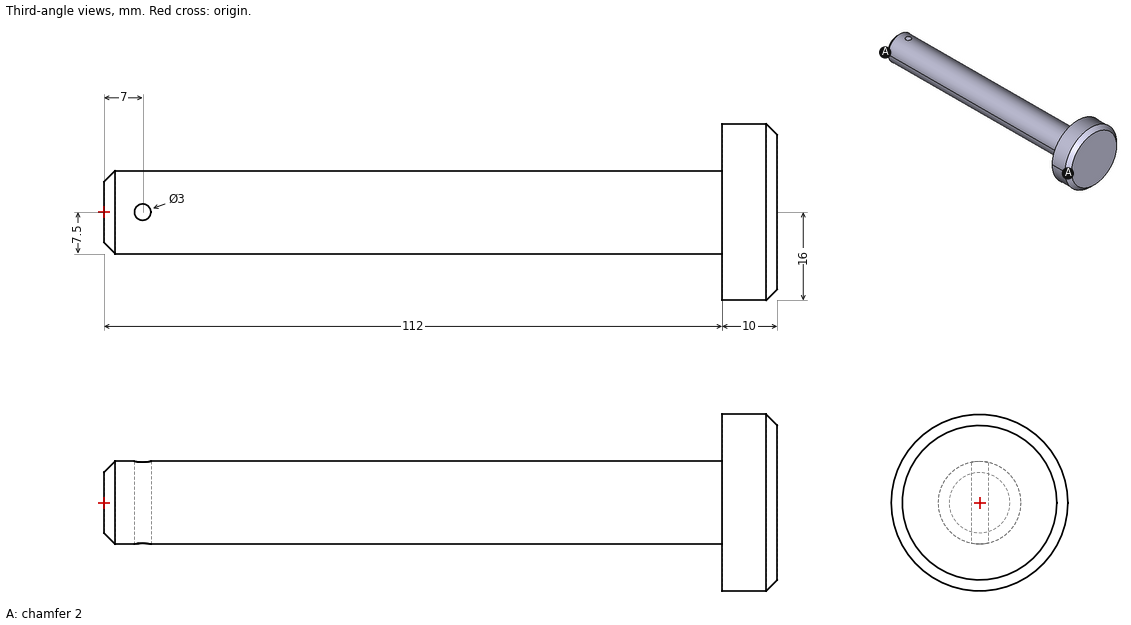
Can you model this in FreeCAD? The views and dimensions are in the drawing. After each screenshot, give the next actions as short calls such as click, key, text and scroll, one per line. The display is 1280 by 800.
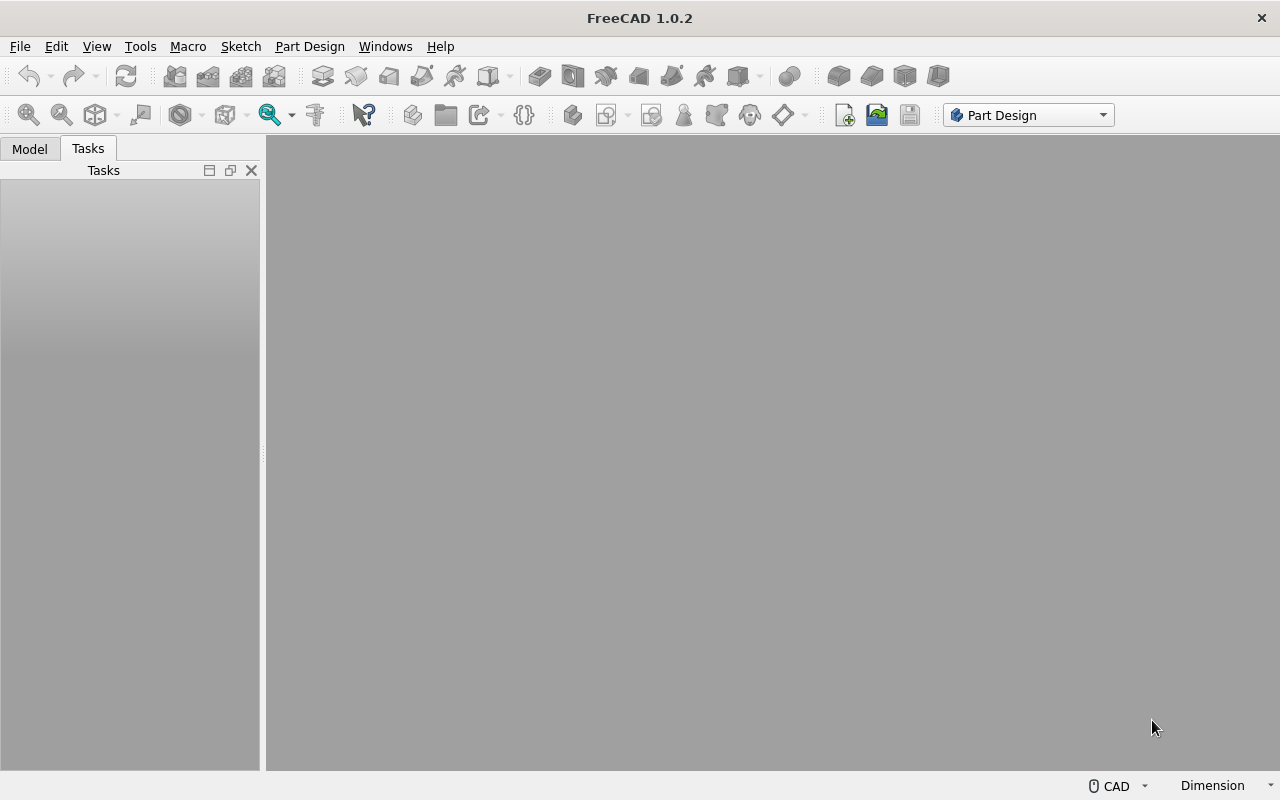
click(844, 116)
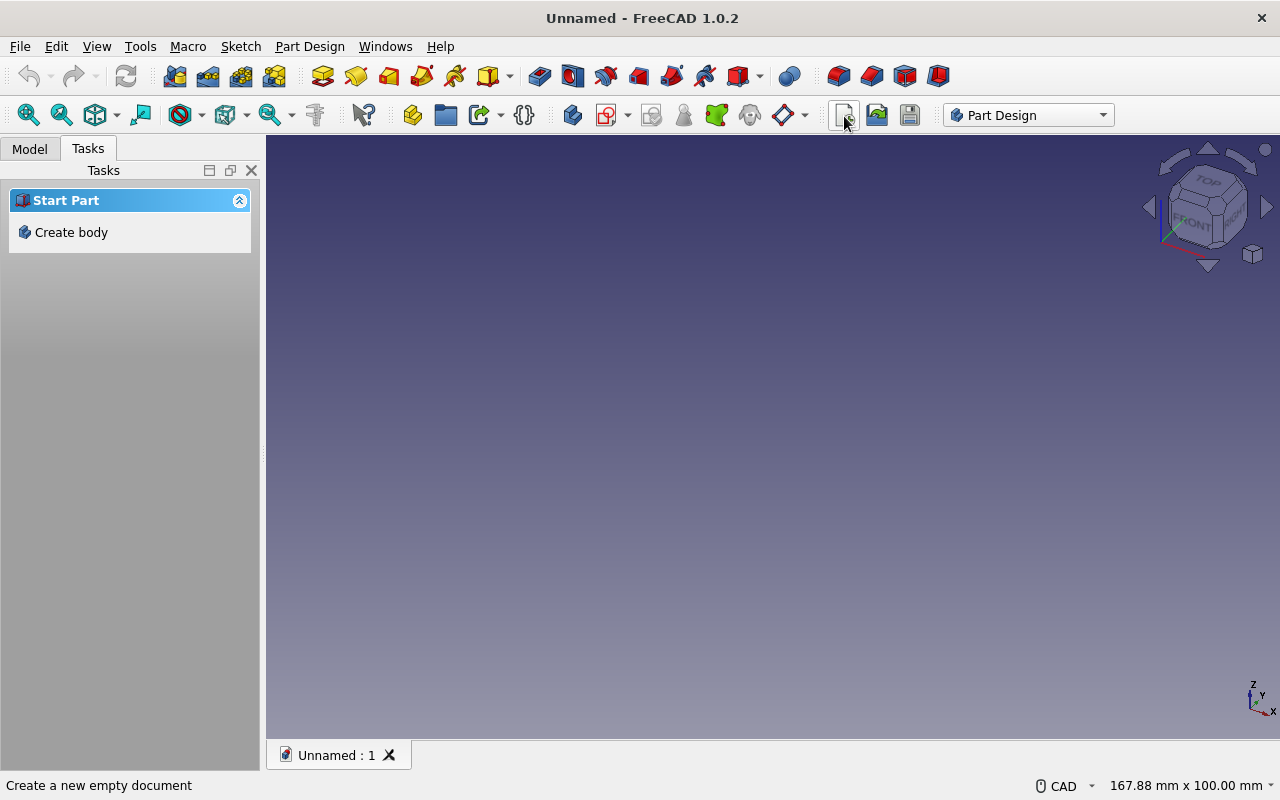
click(606, 116)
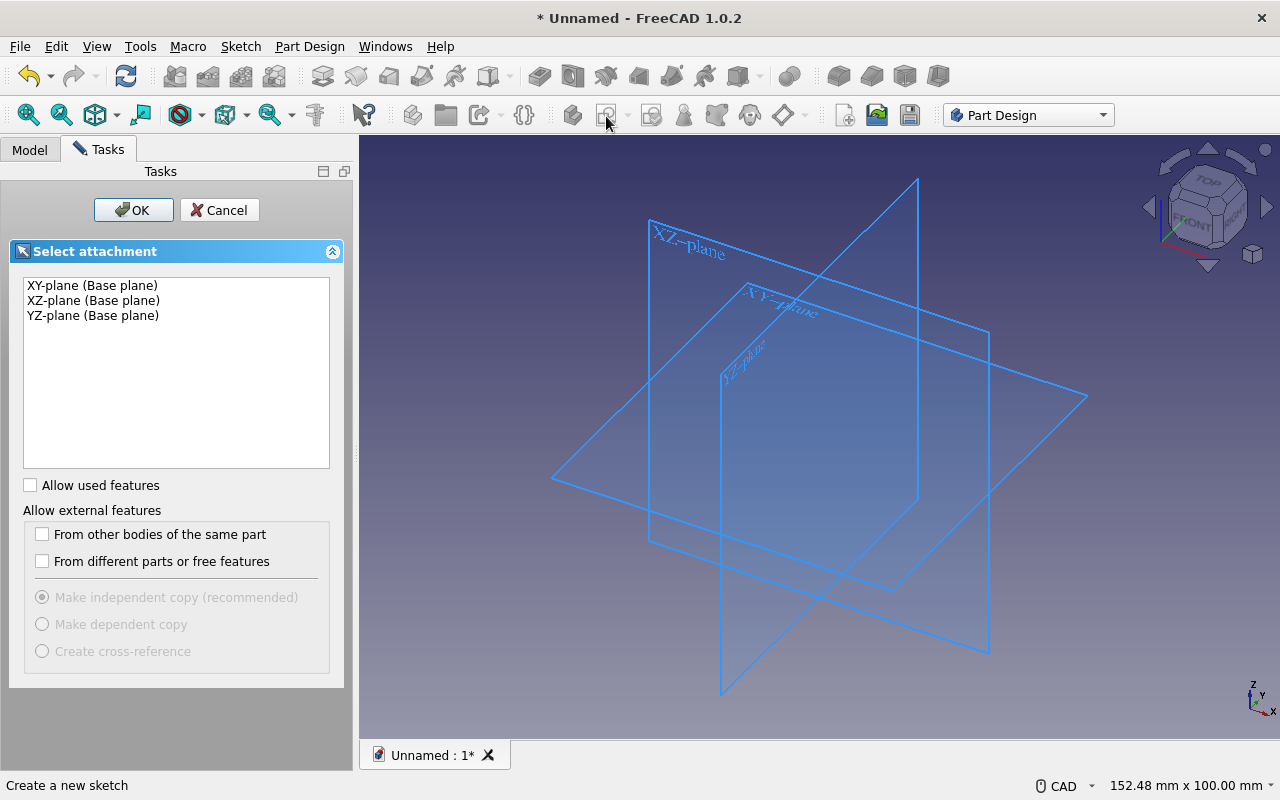
click(84, 286)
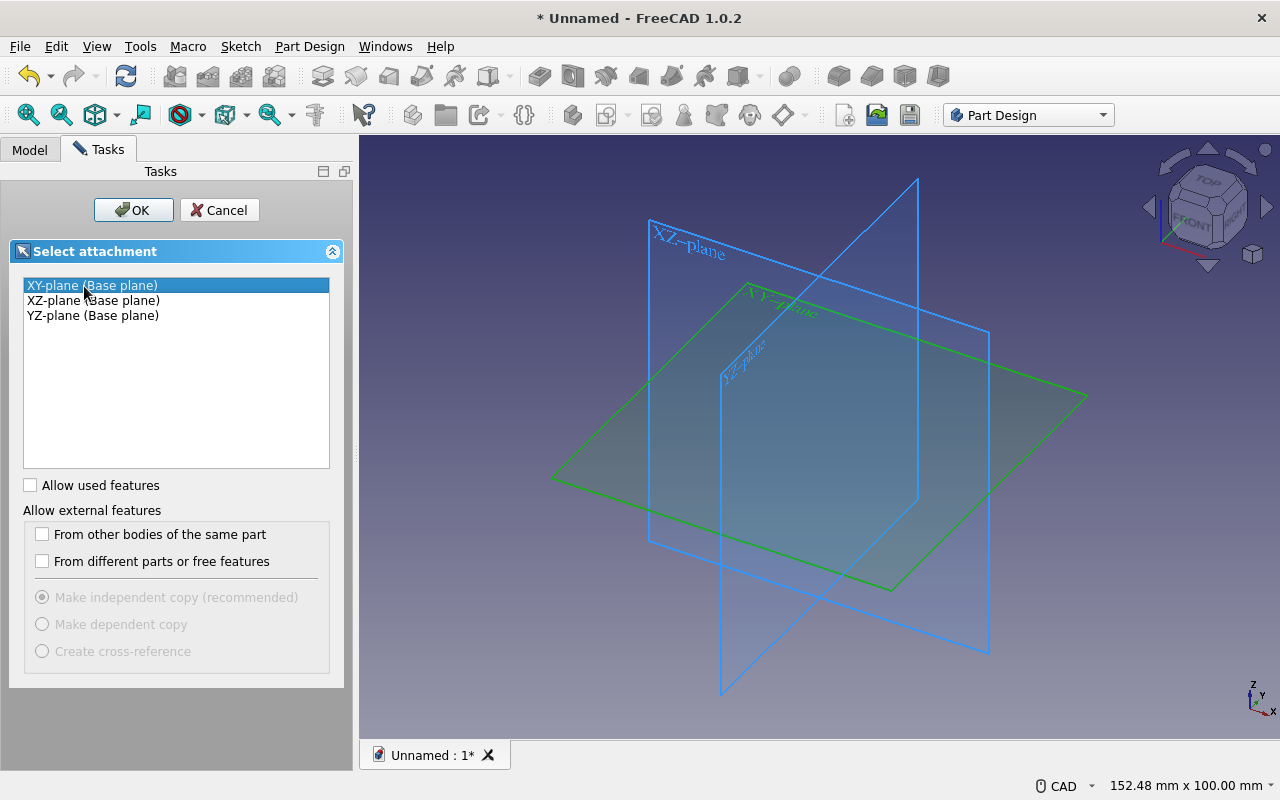
click(134, 210)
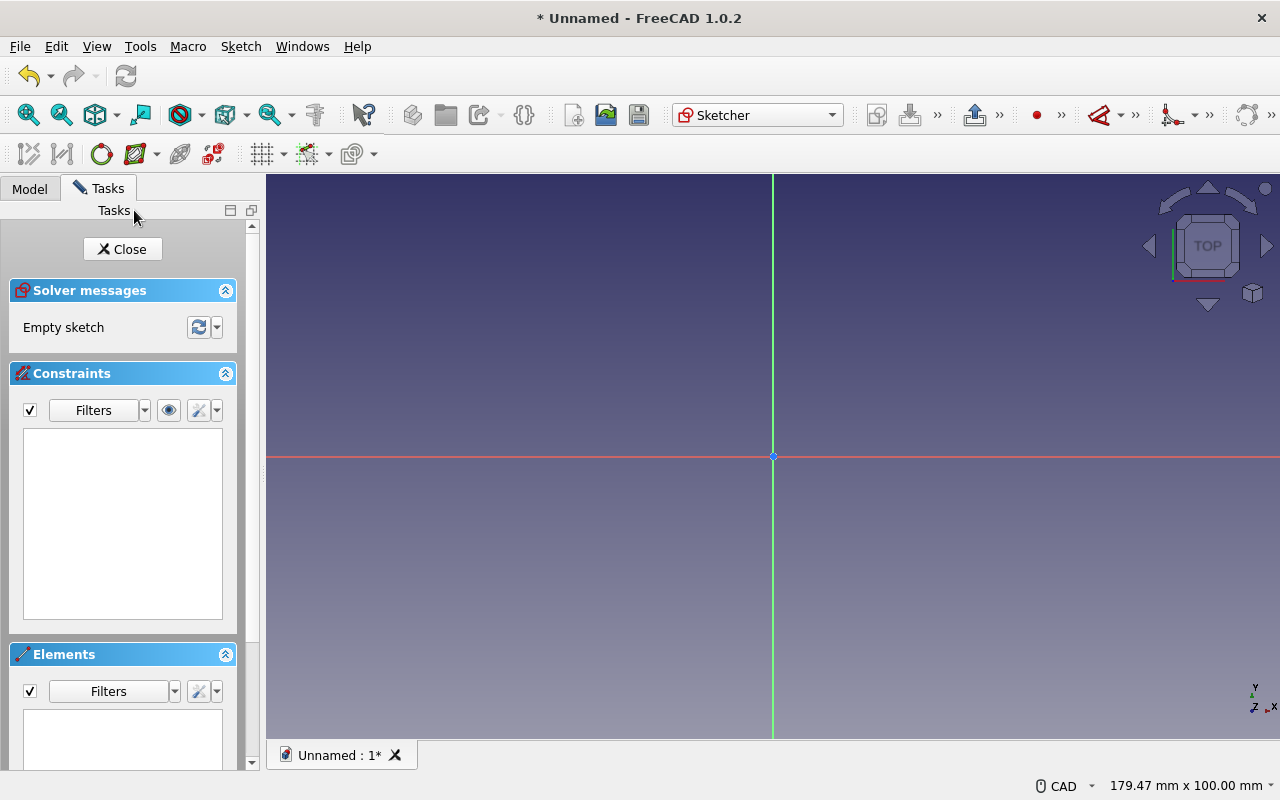
scroll(294, 365, down, 2)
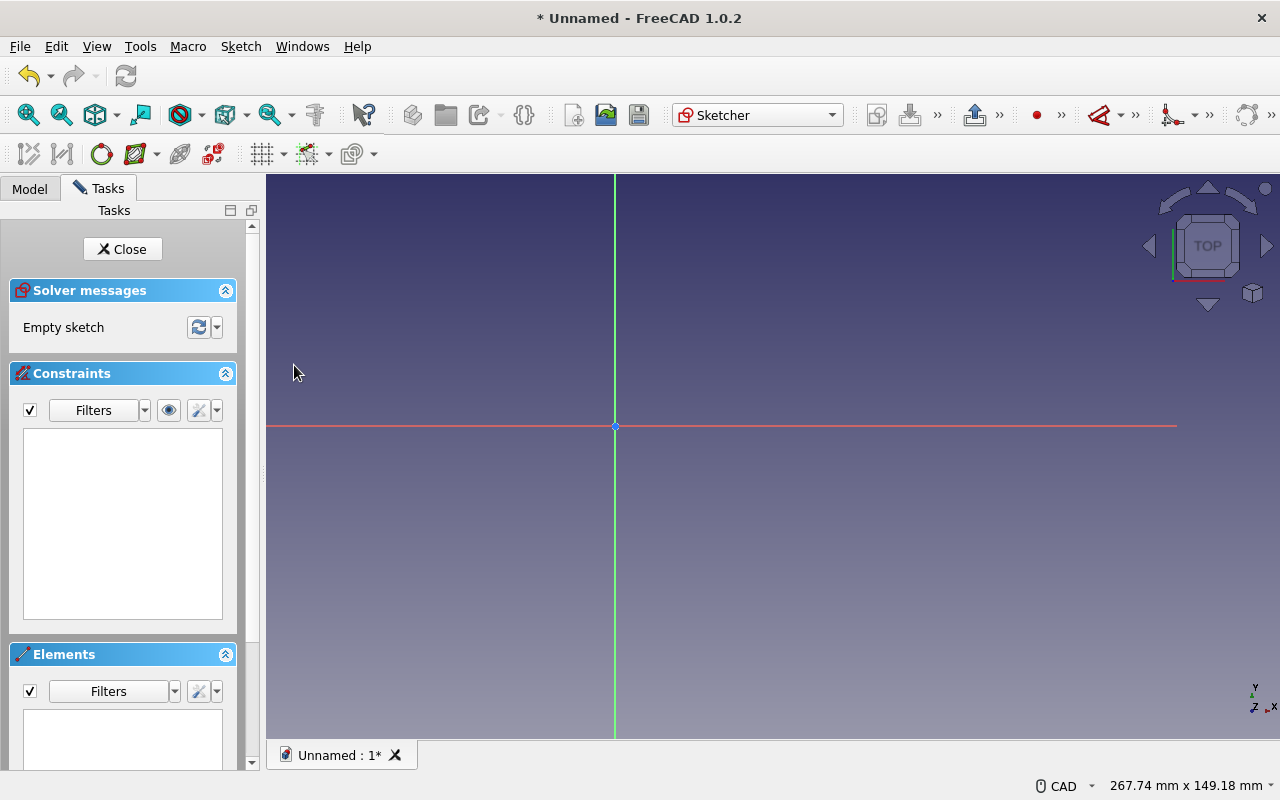
key(g)
key(m)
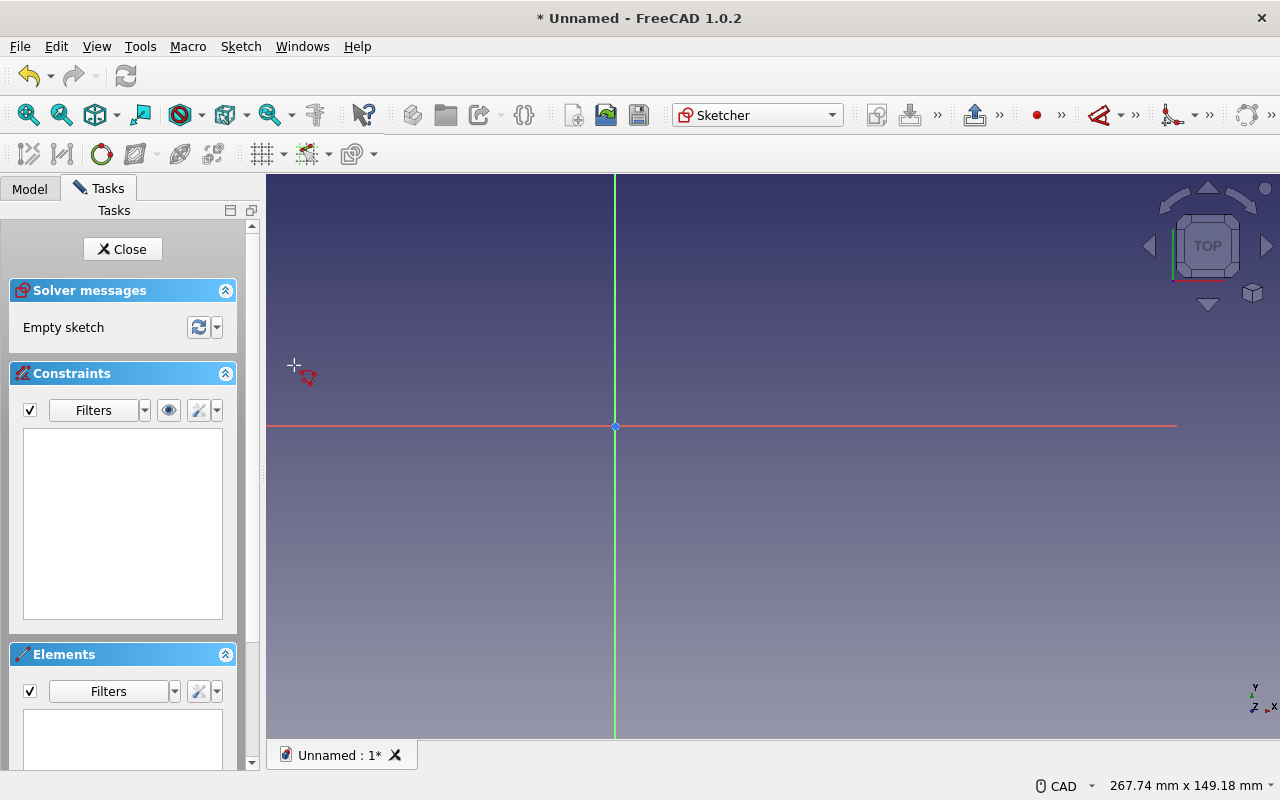
click(615, 426)
click(624, 455)
click(1039, 455)
click(1039, 487)
click(1077, 487)
click(1077, 435)
click(615, 426)
key(Escape)
key(Escape)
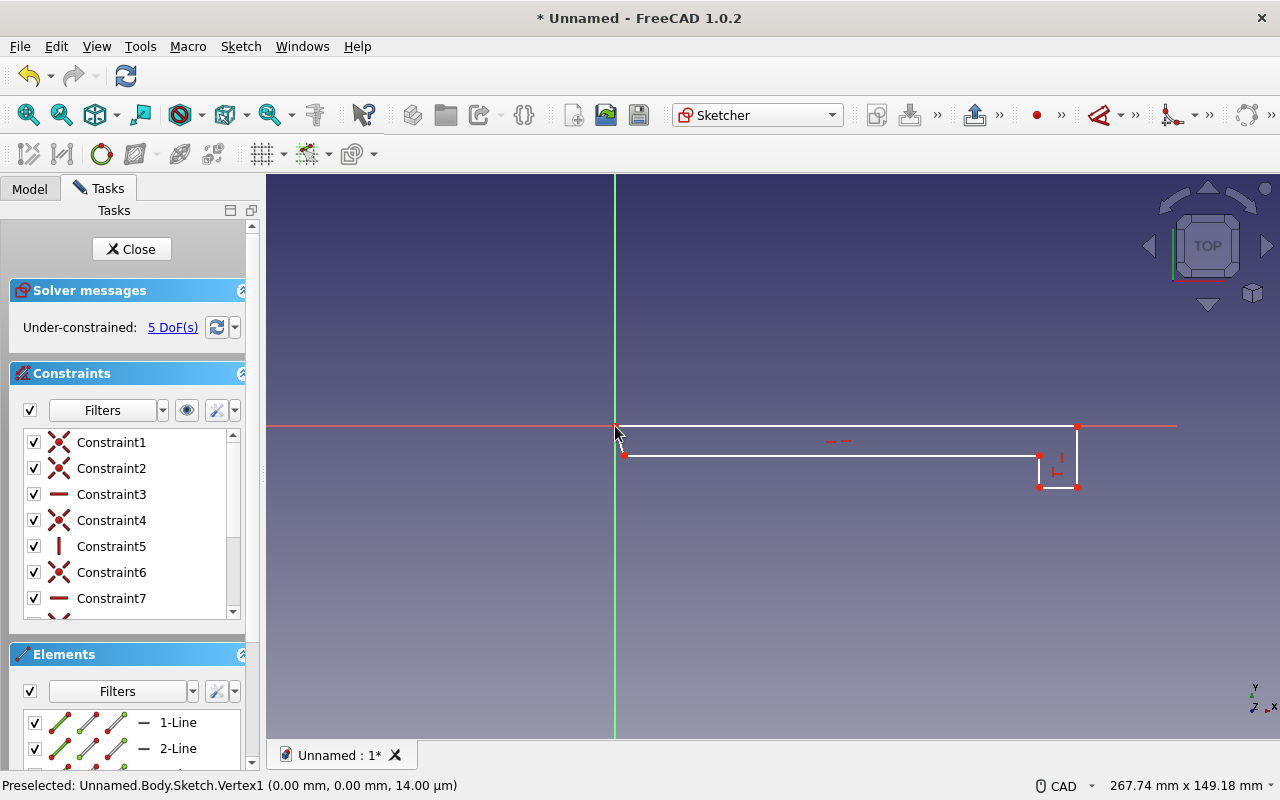
click(619, 438)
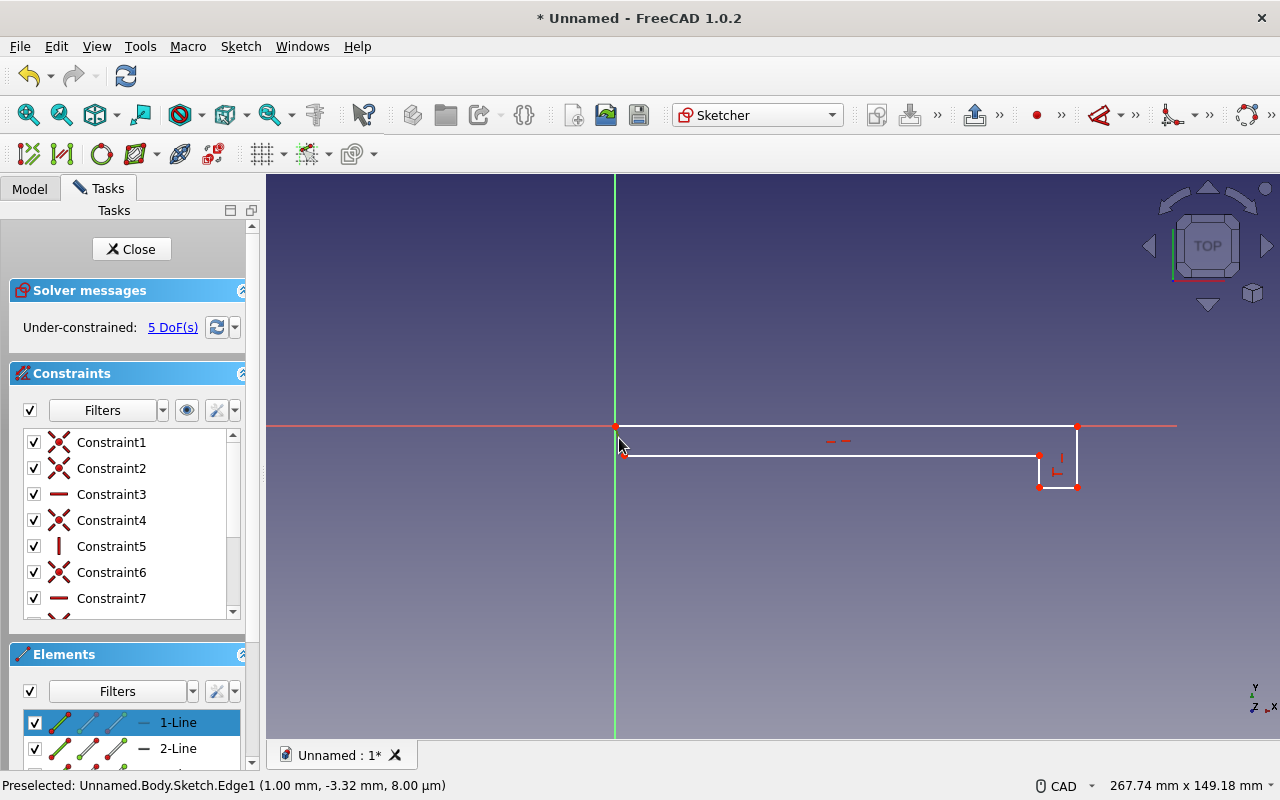
key(v)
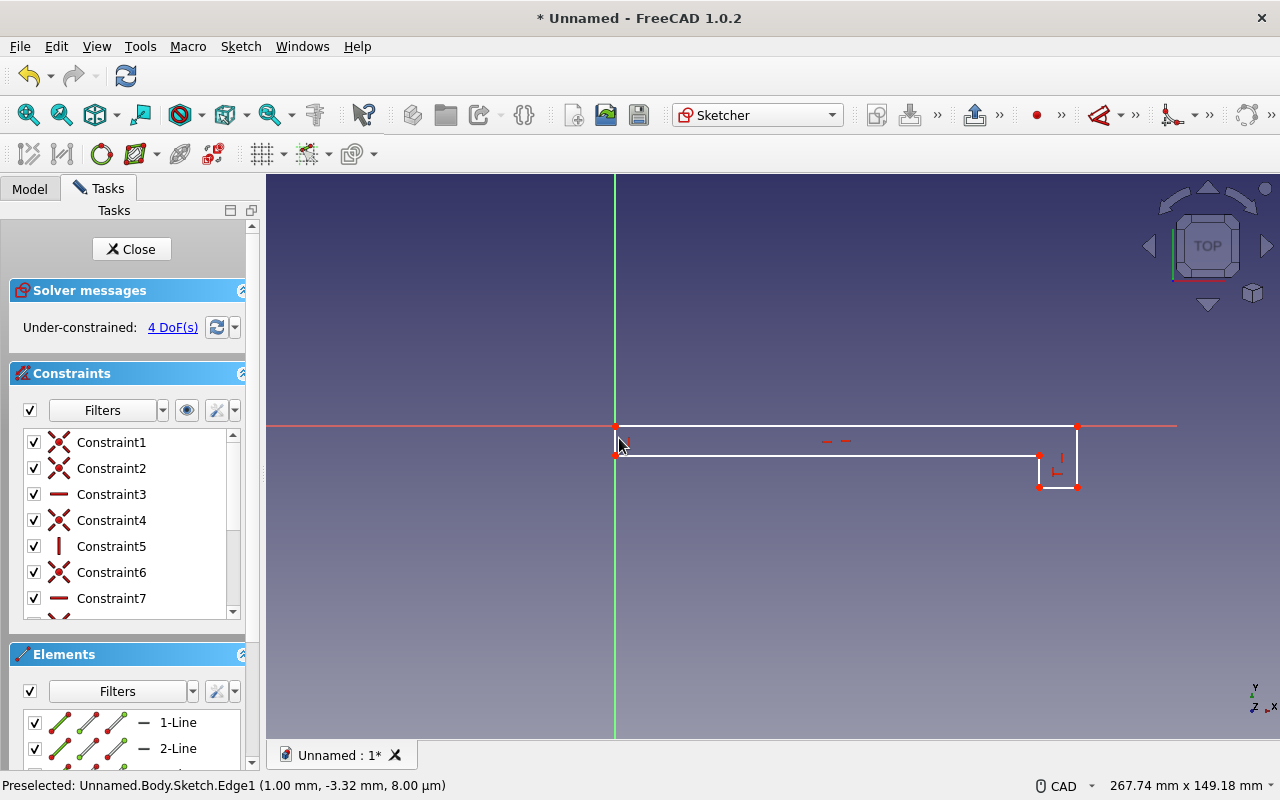
click(1050, 488)